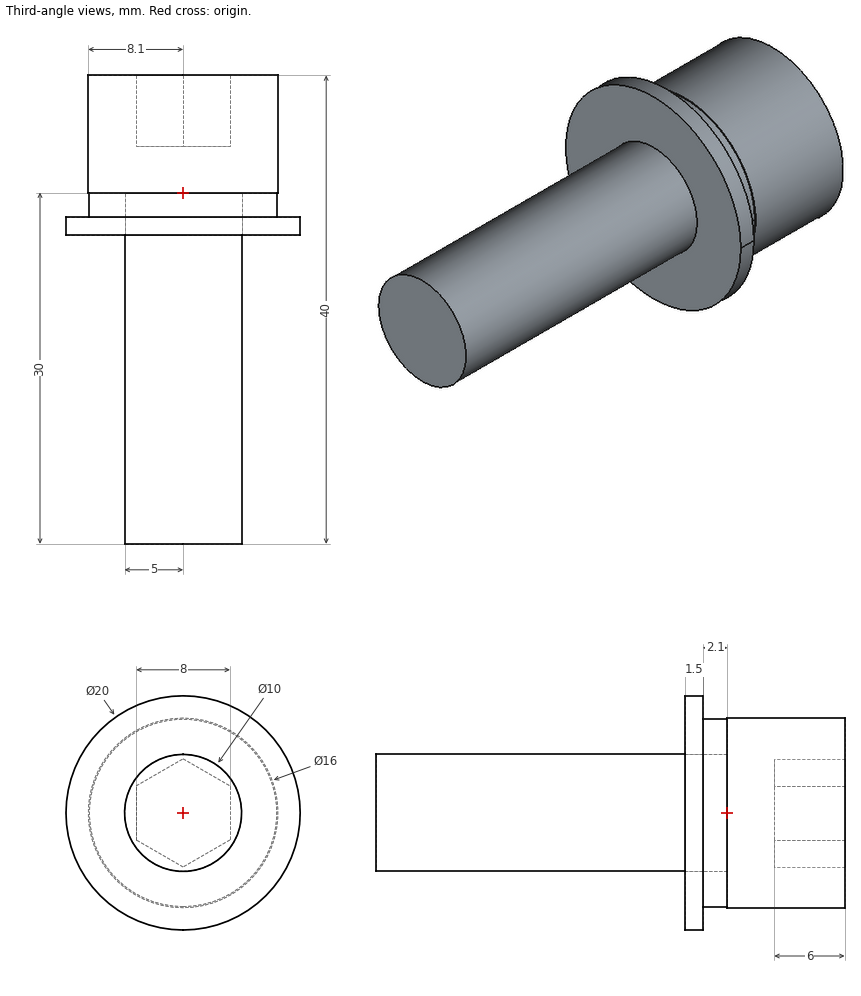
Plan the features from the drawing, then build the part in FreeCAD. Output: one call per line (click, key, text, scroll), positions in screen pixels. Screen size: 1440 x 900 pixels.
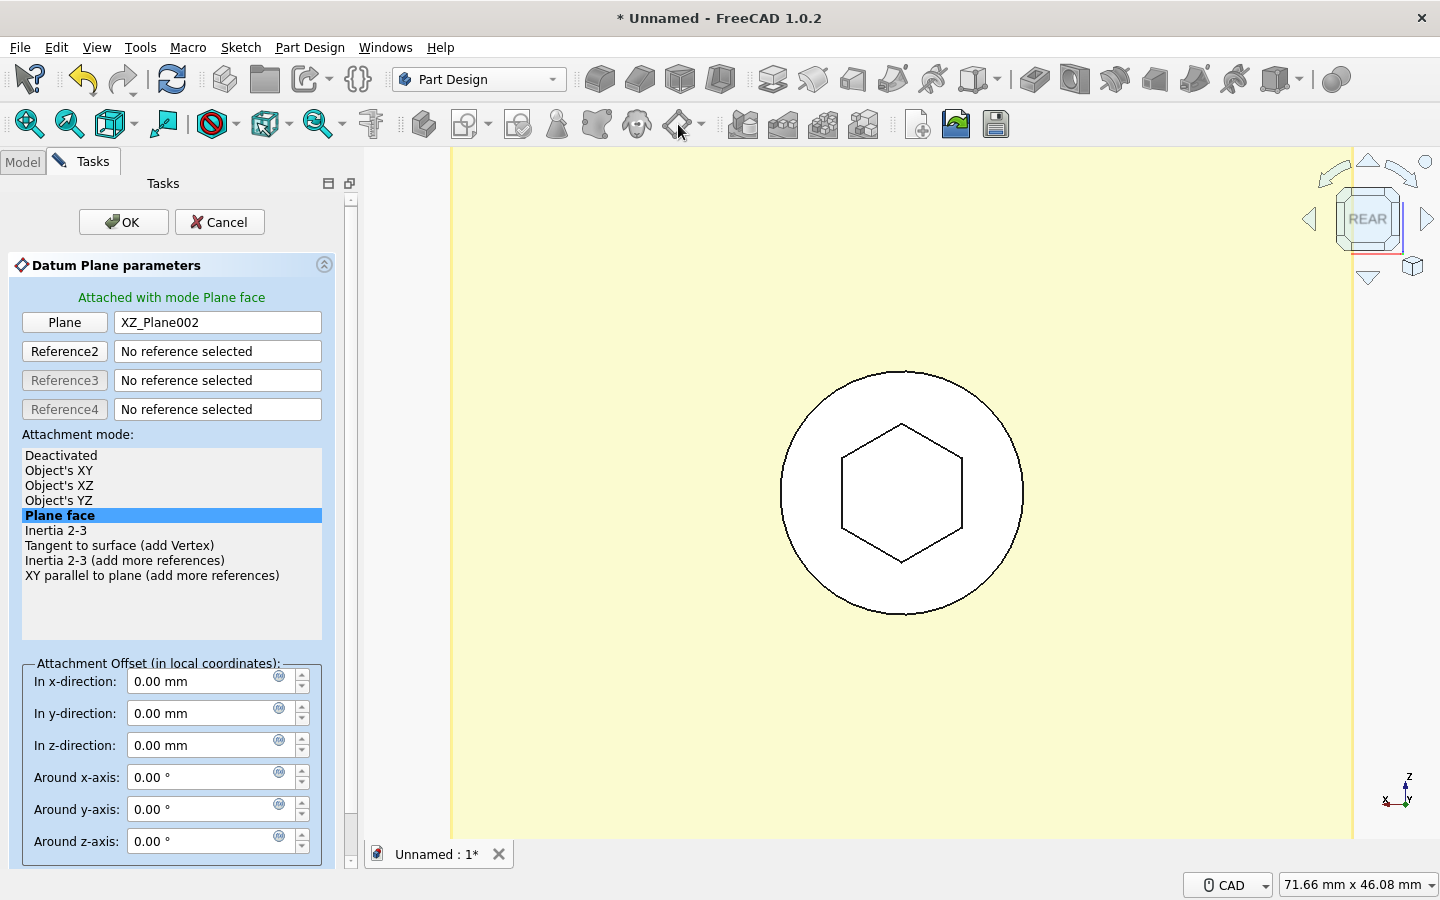
triple_click(210, 745)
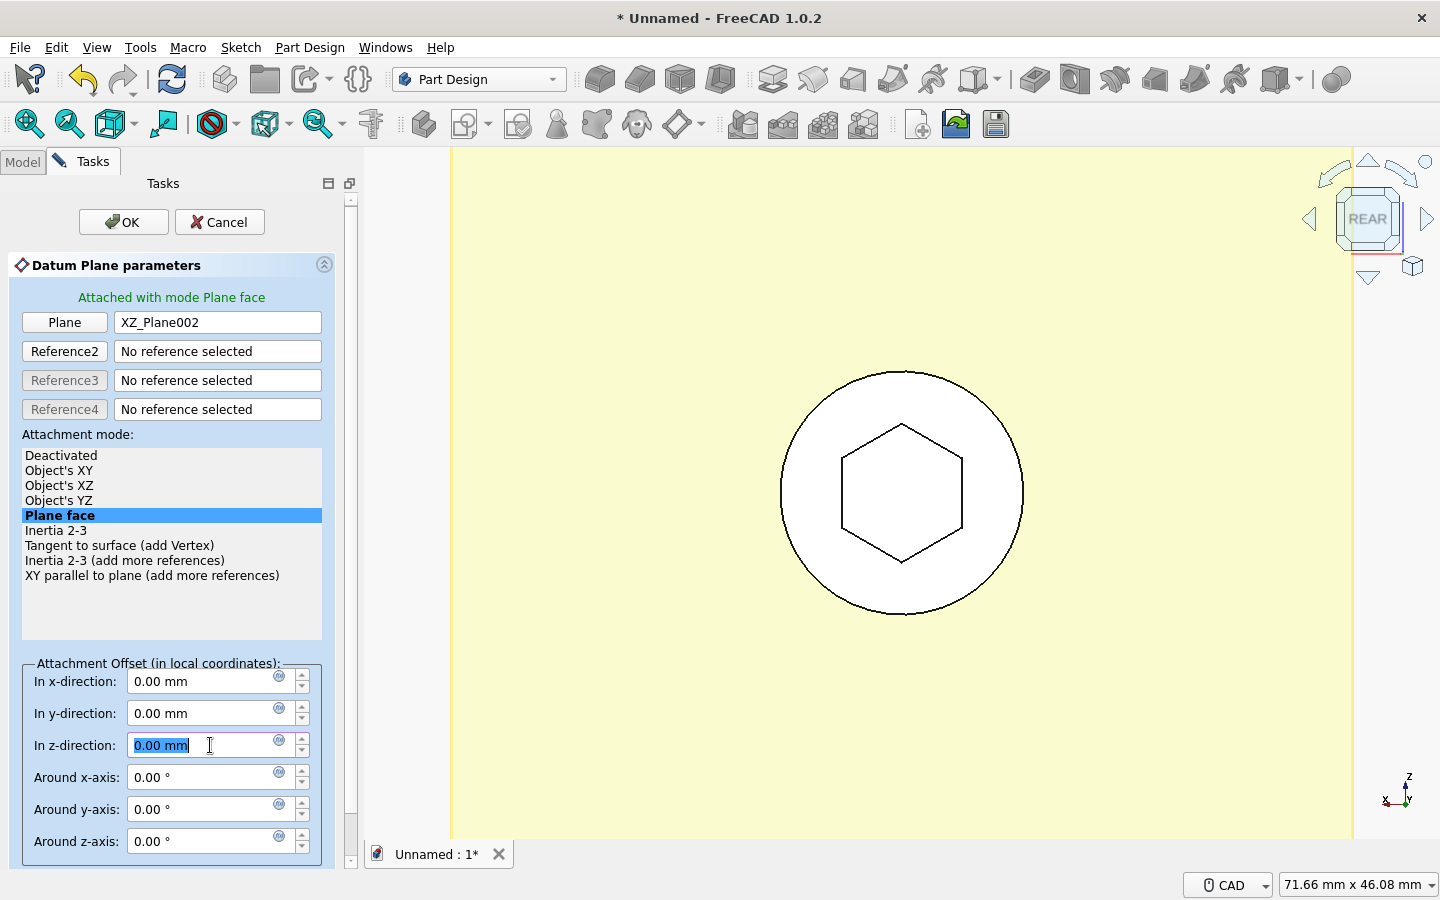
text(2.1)
key(Tab)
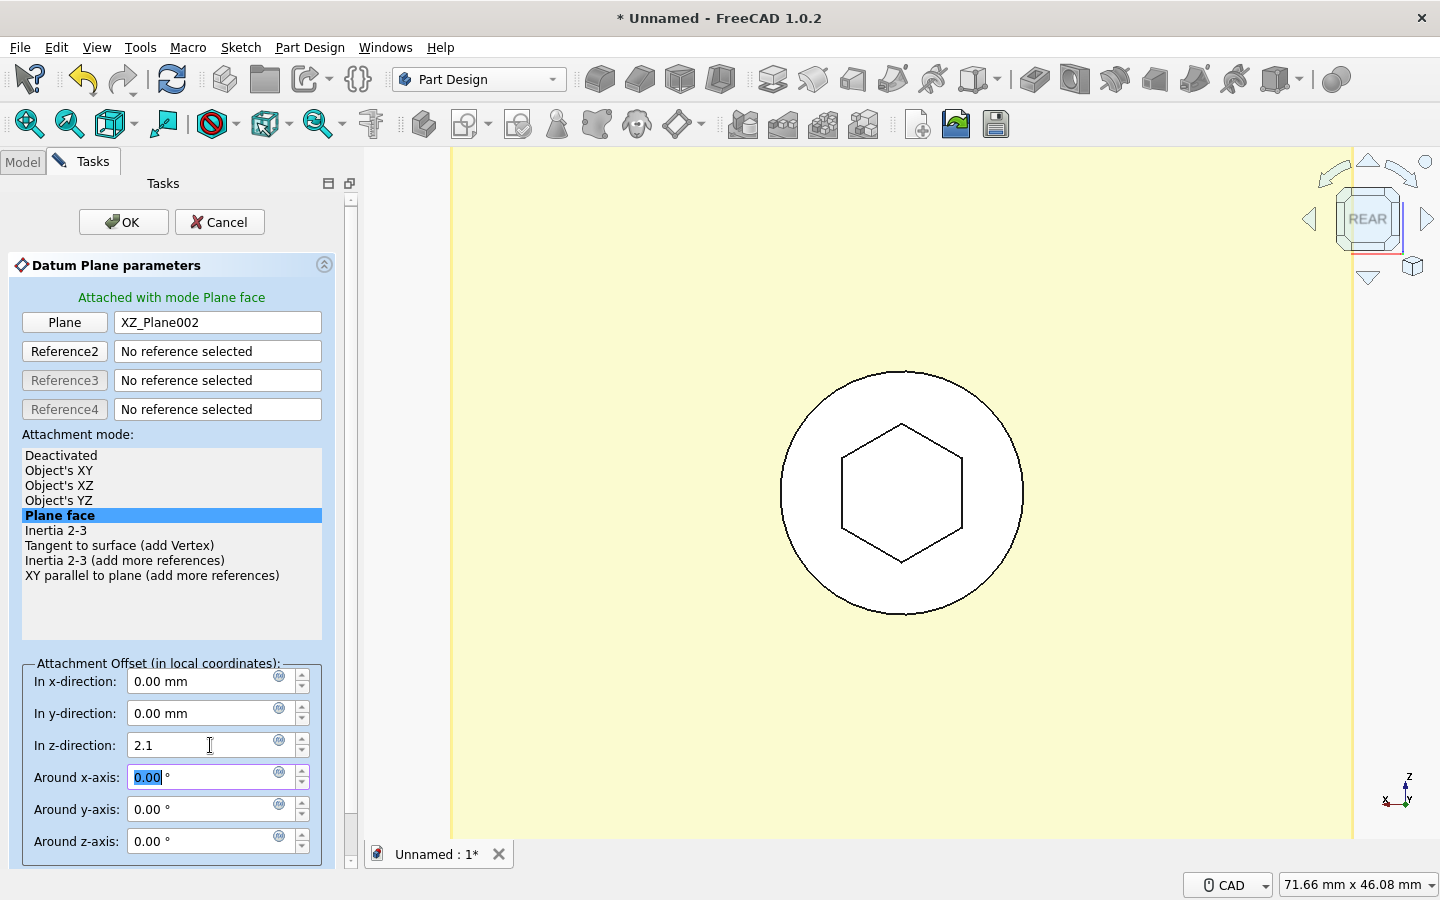
click(124, 222)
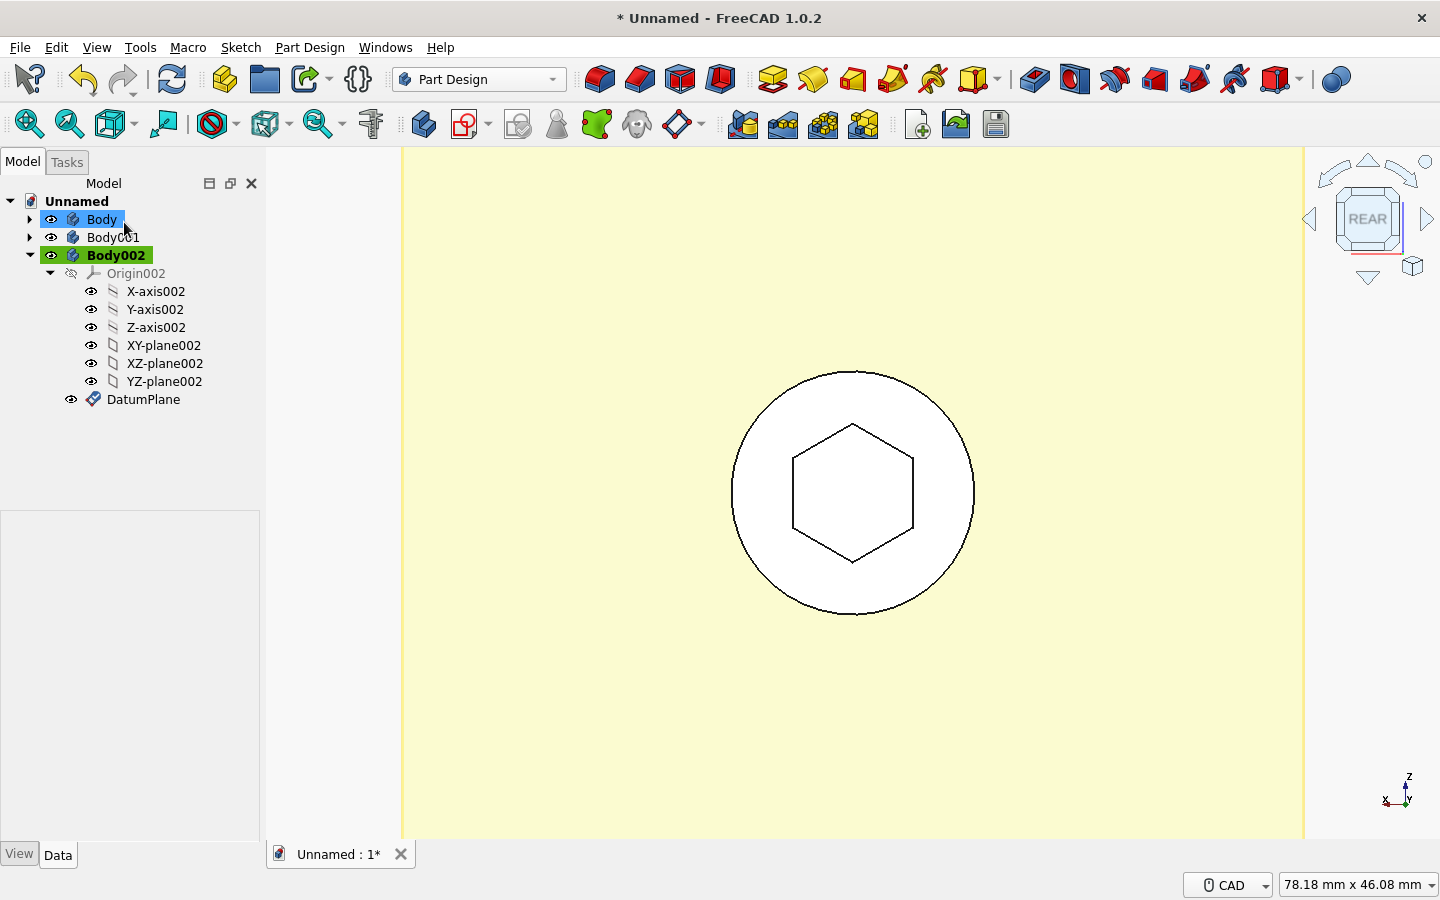
click(116, 399)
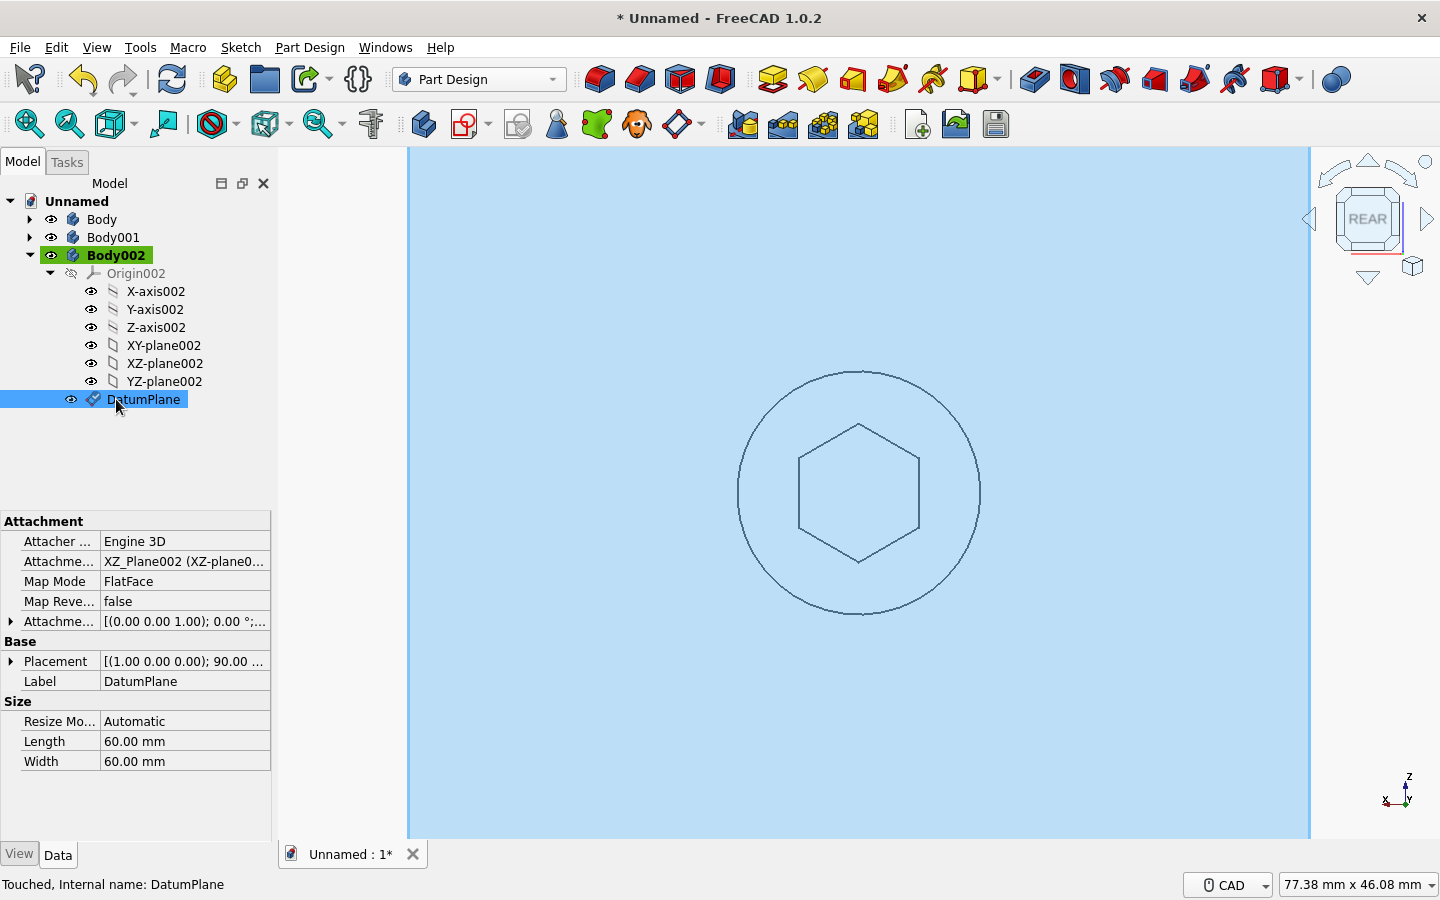
click(464, 124)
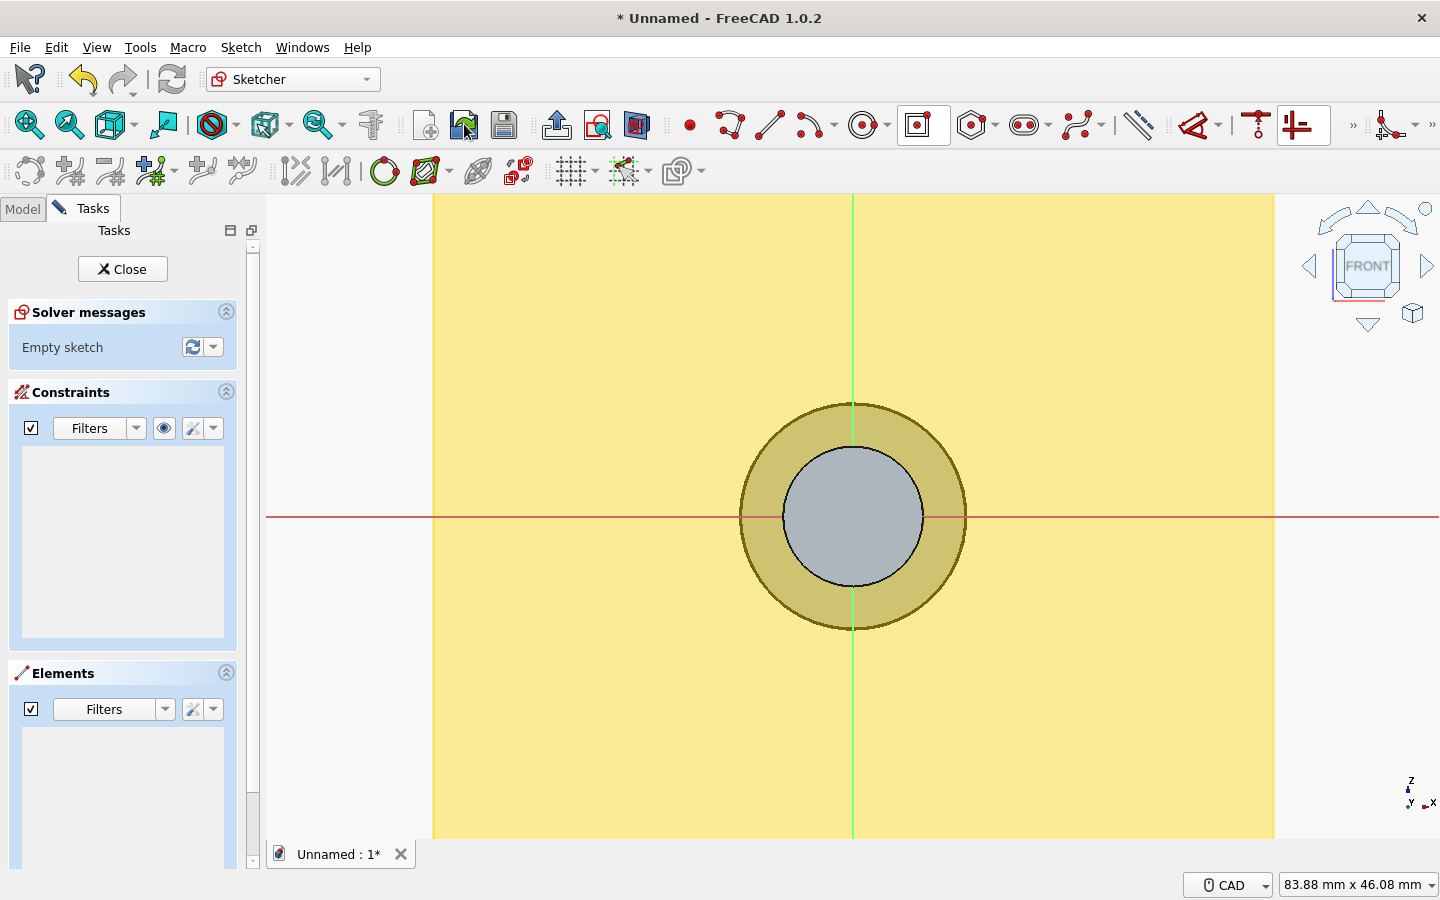
scroll(993, 517, up, 2)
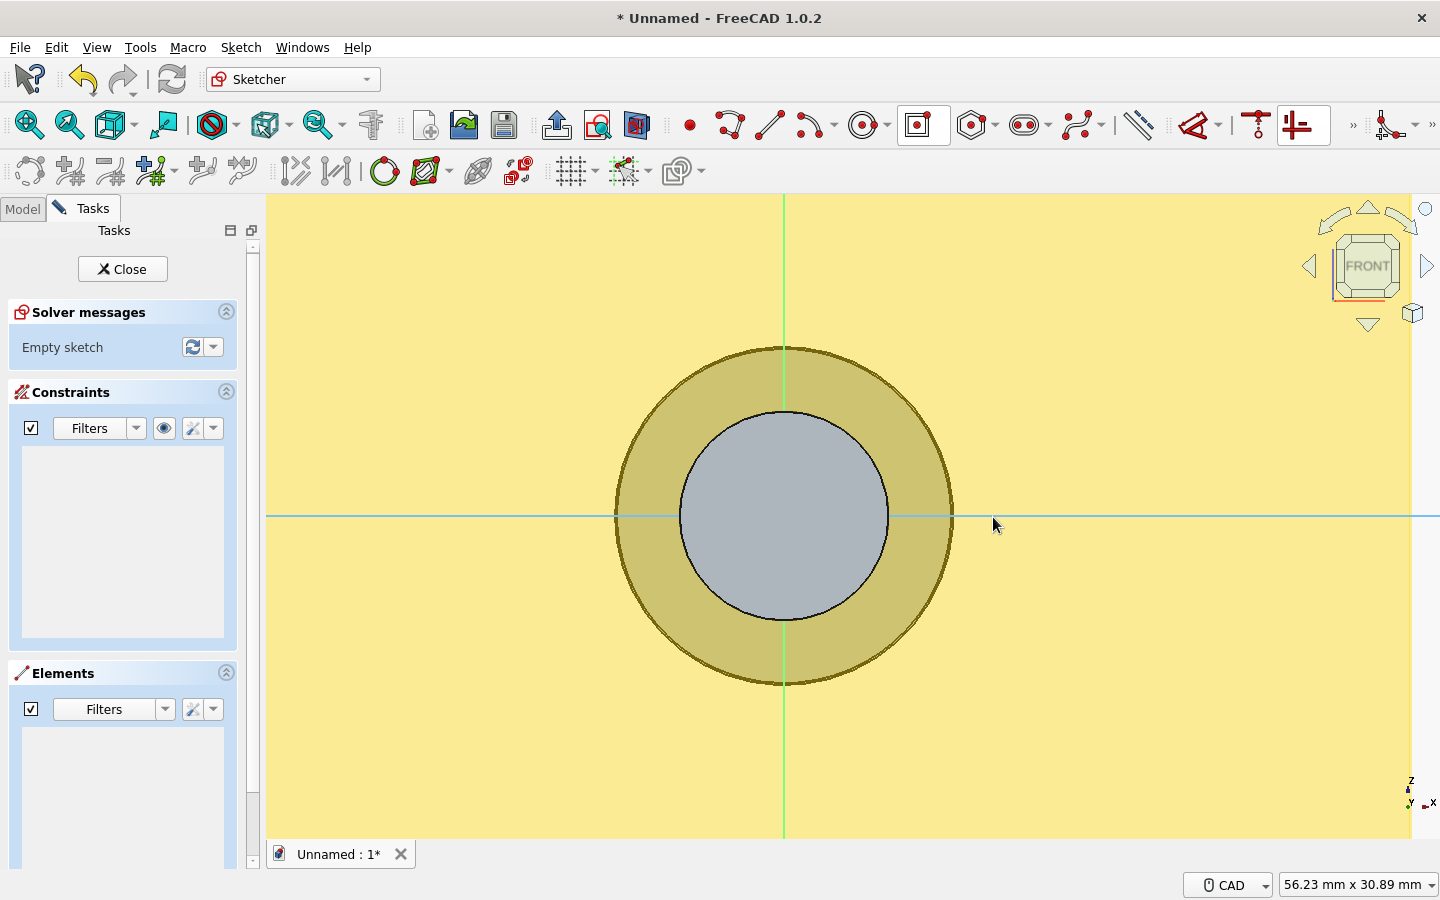
click(864, 126)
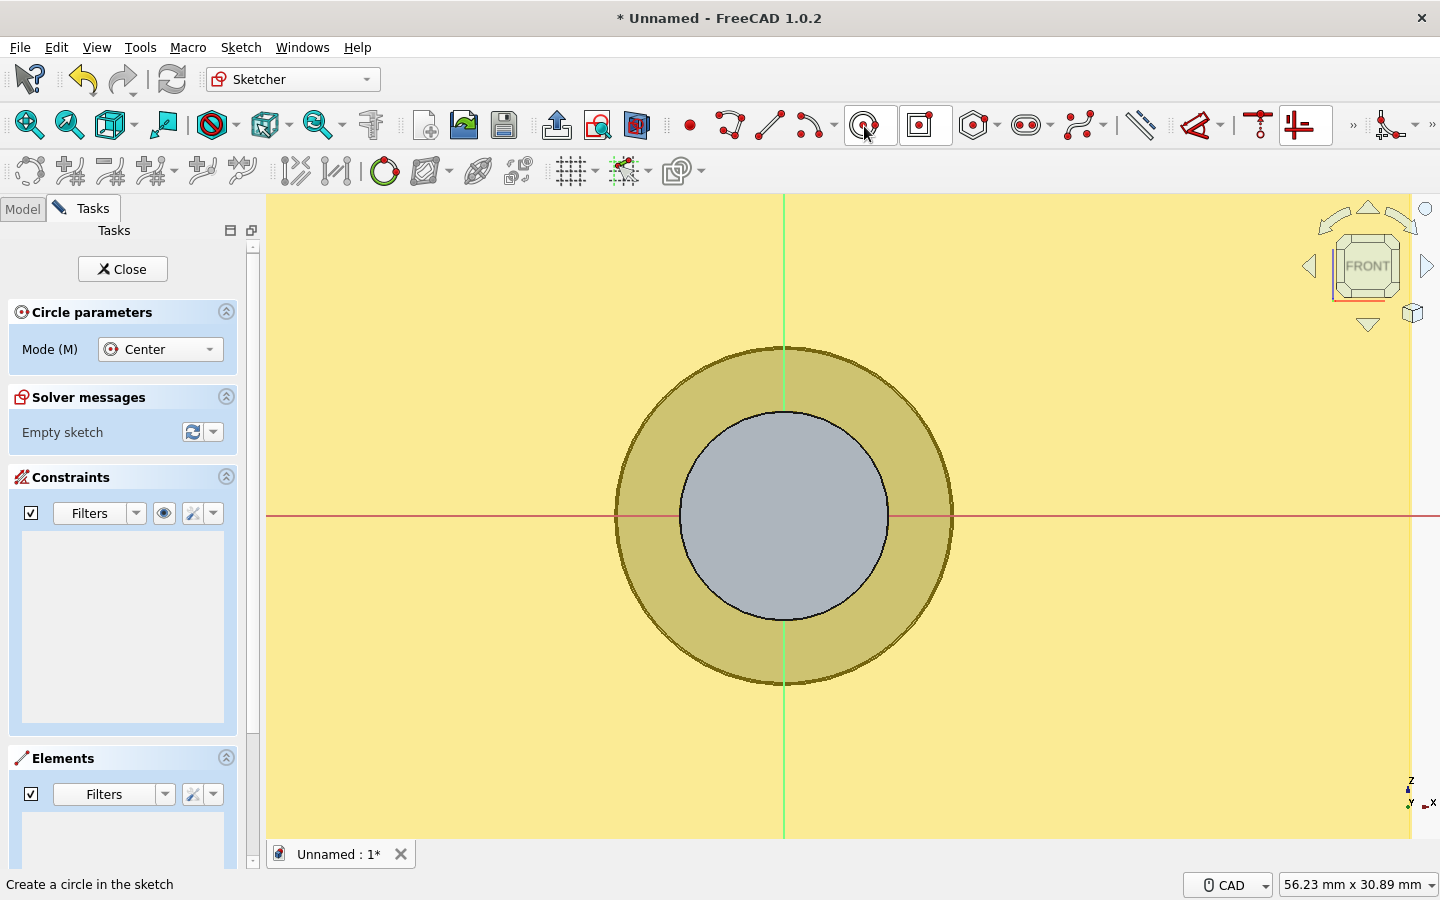
click(784, 516)
move(932, 368)